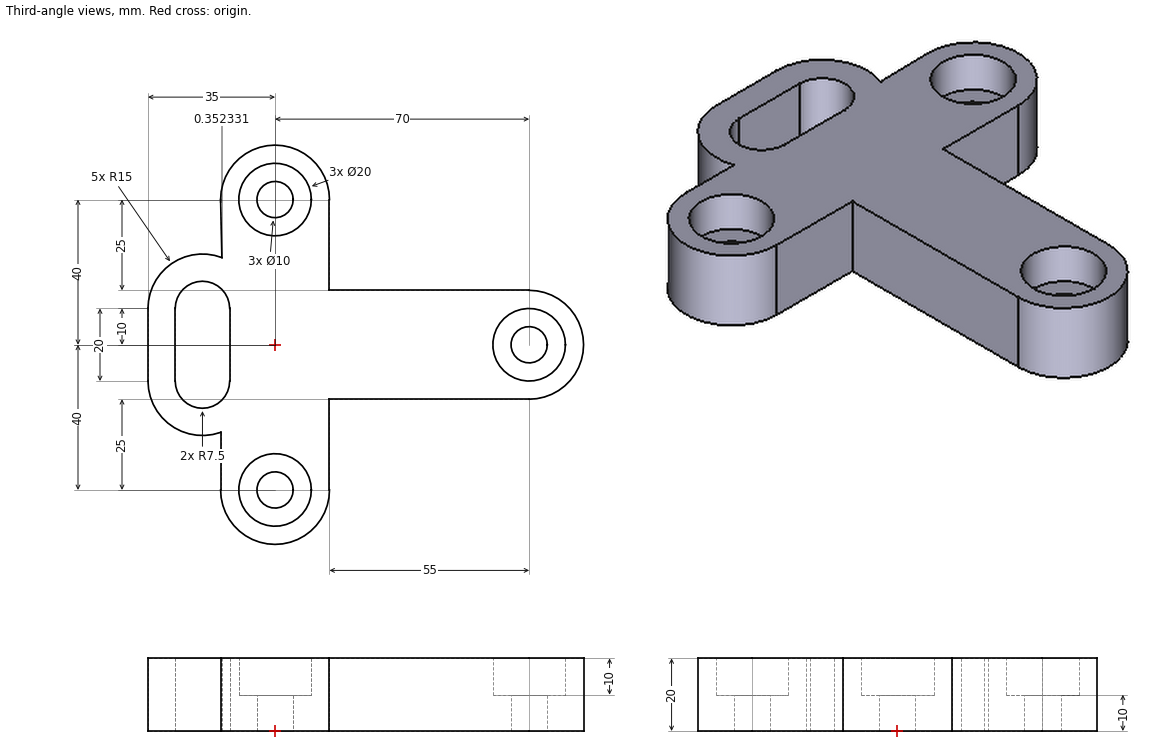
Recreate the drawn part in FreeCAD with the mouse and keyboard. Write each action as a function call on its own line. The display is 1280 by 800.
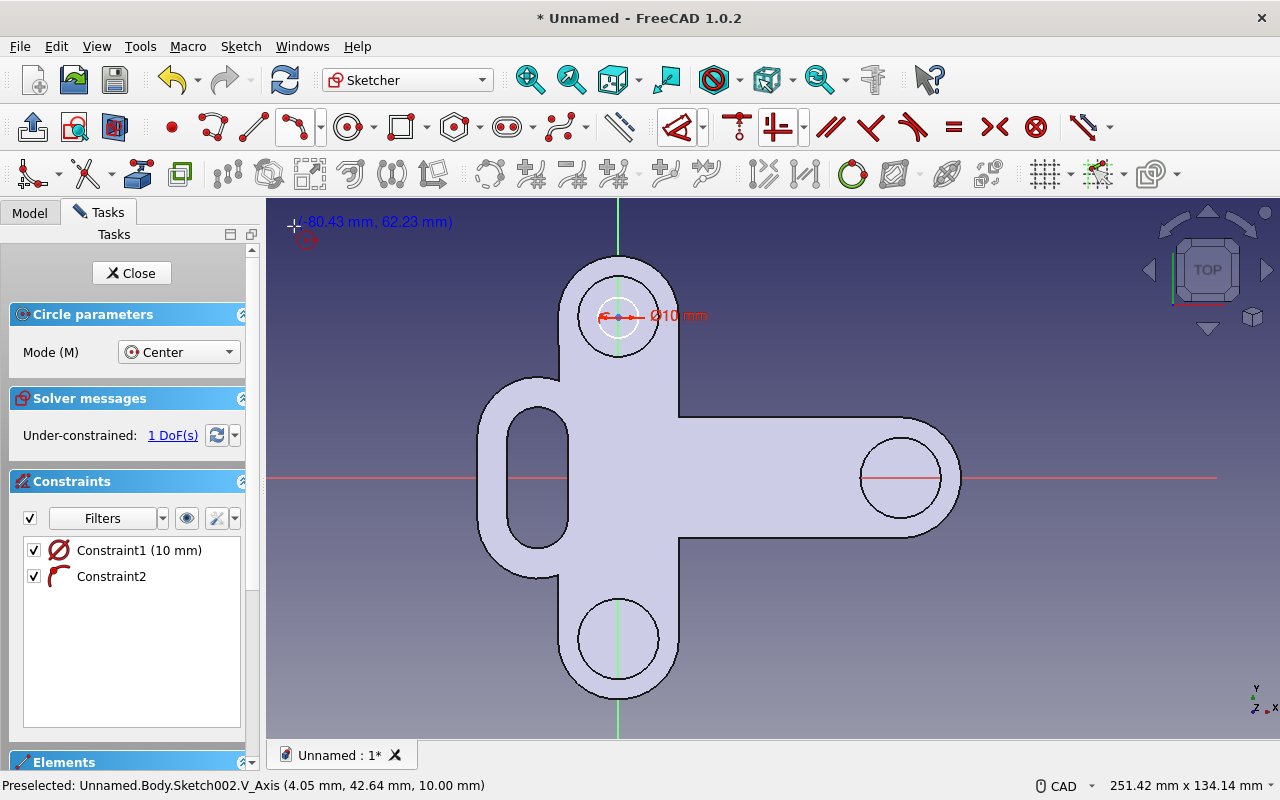
click(618, 639)
move(633, 625)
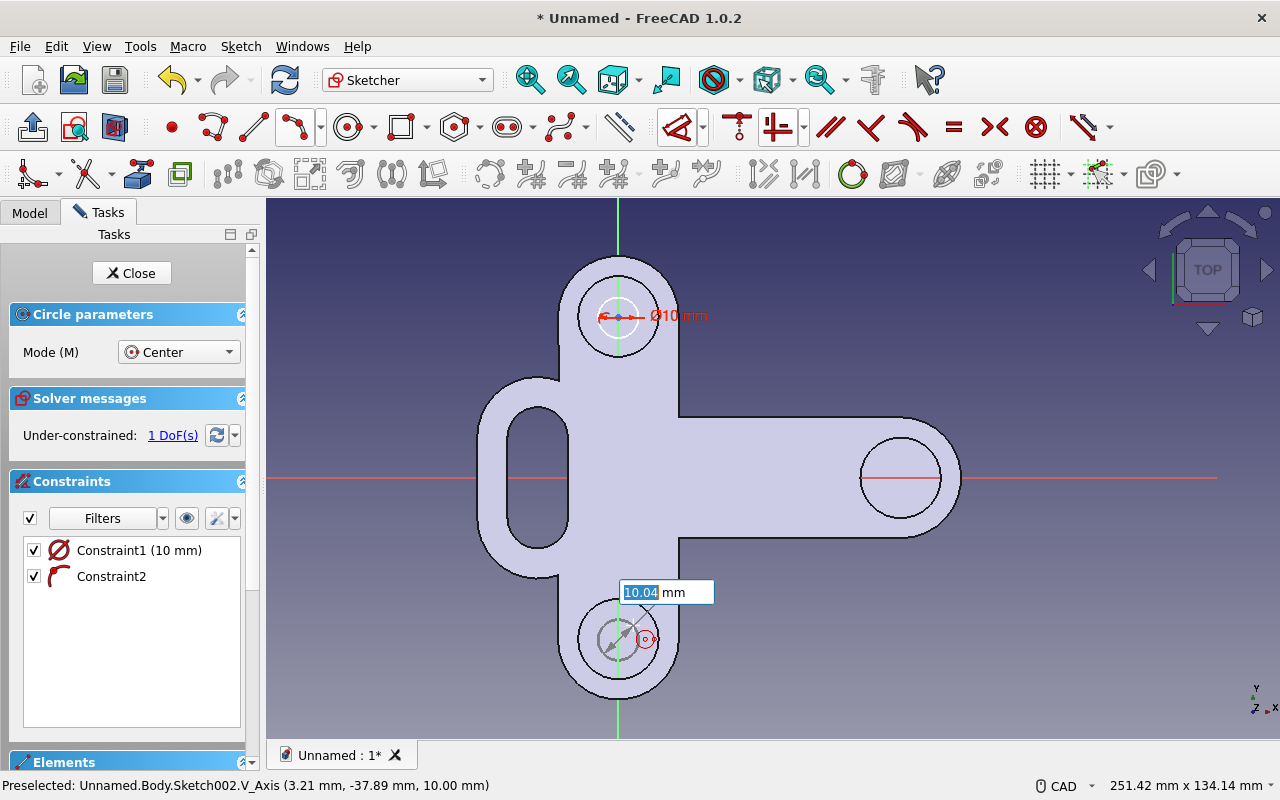
text(10)
key(Return)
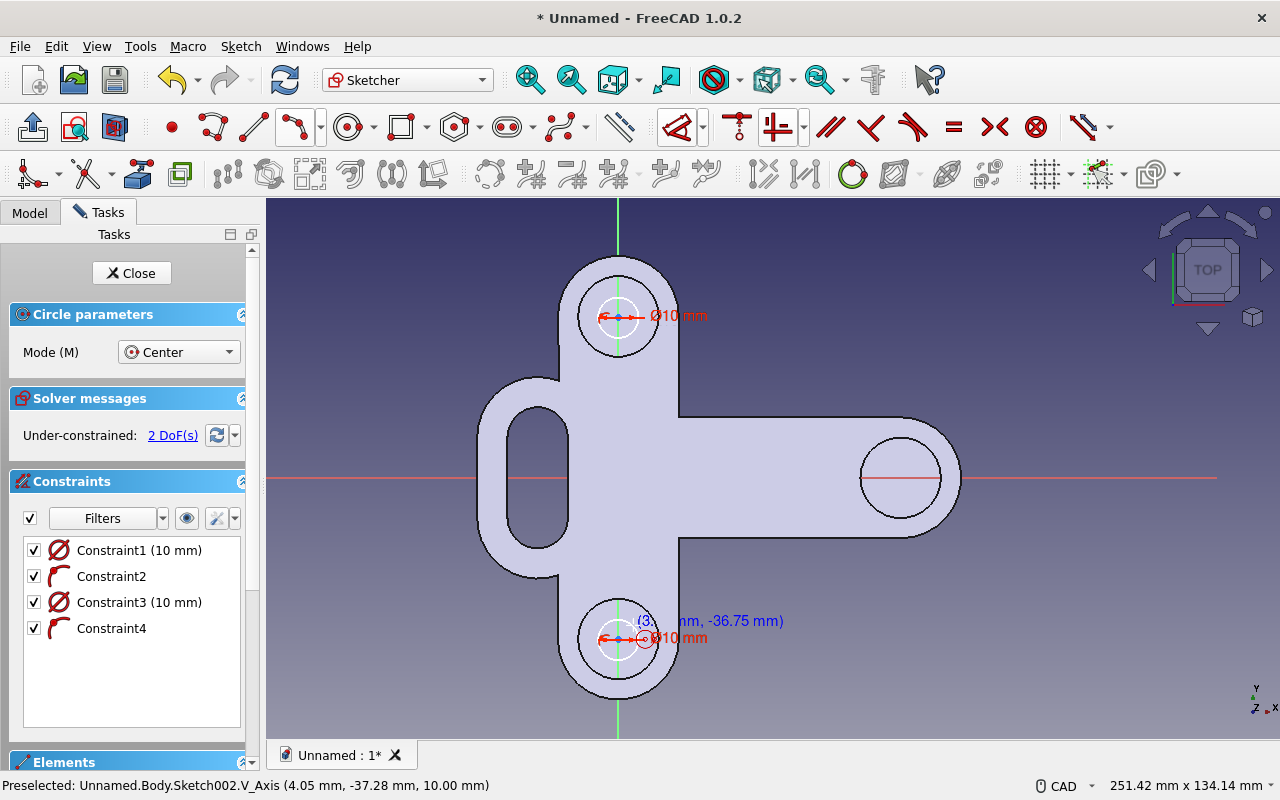
click(901, 478)
move(915, 464)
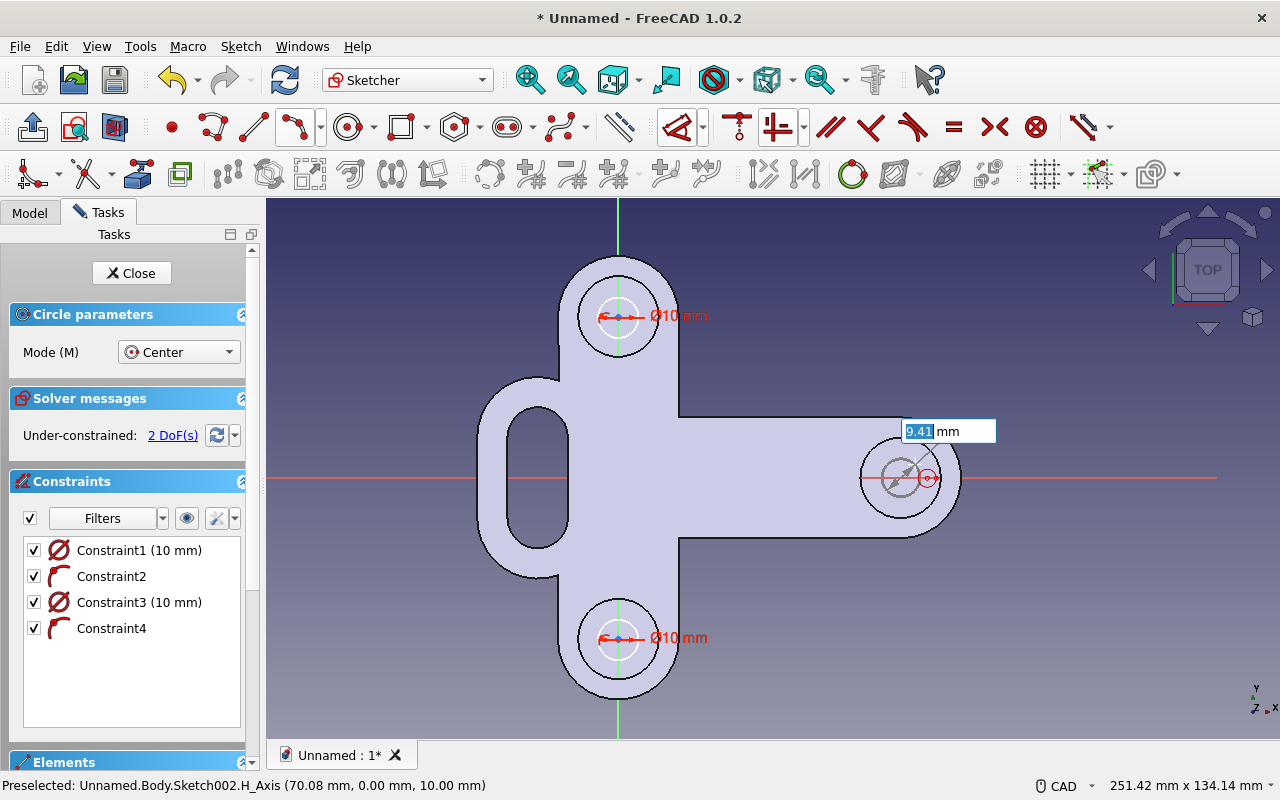
text(10)
key(Return)
key(Escape)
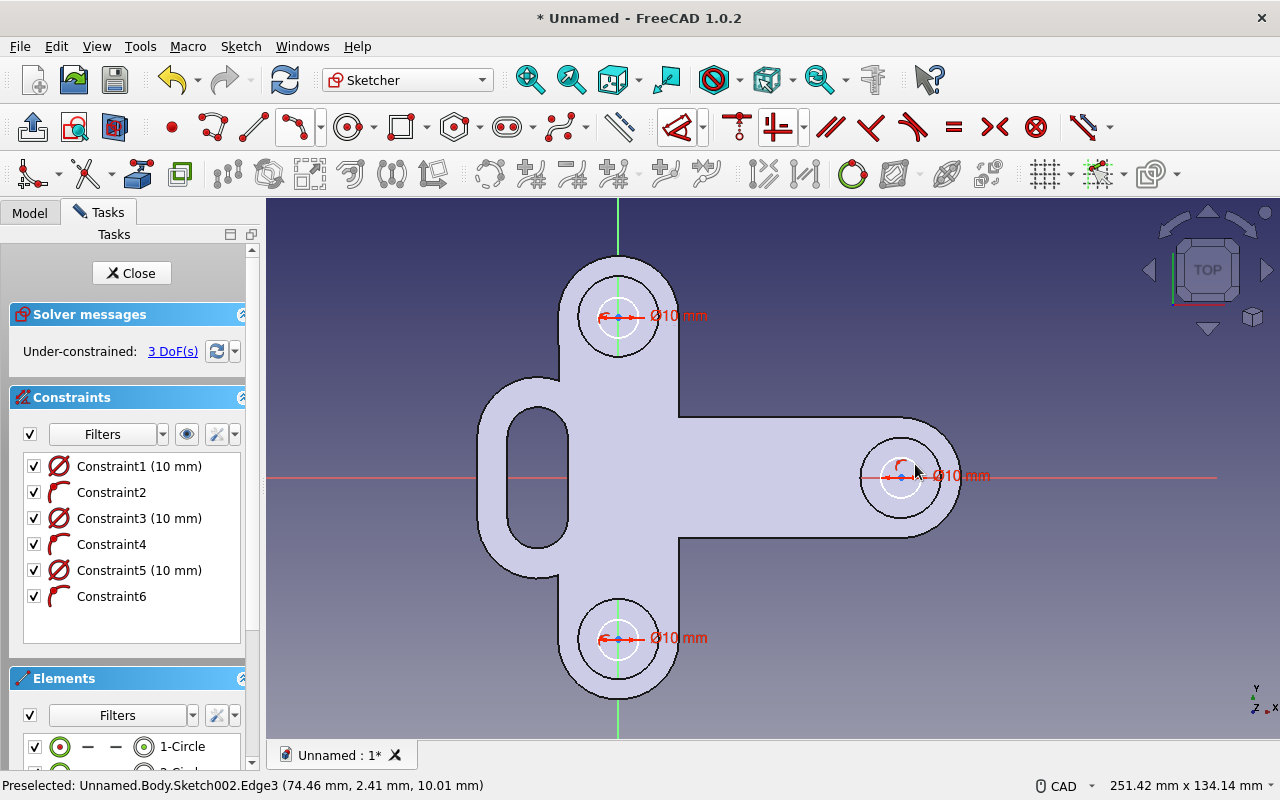
click(618, 318)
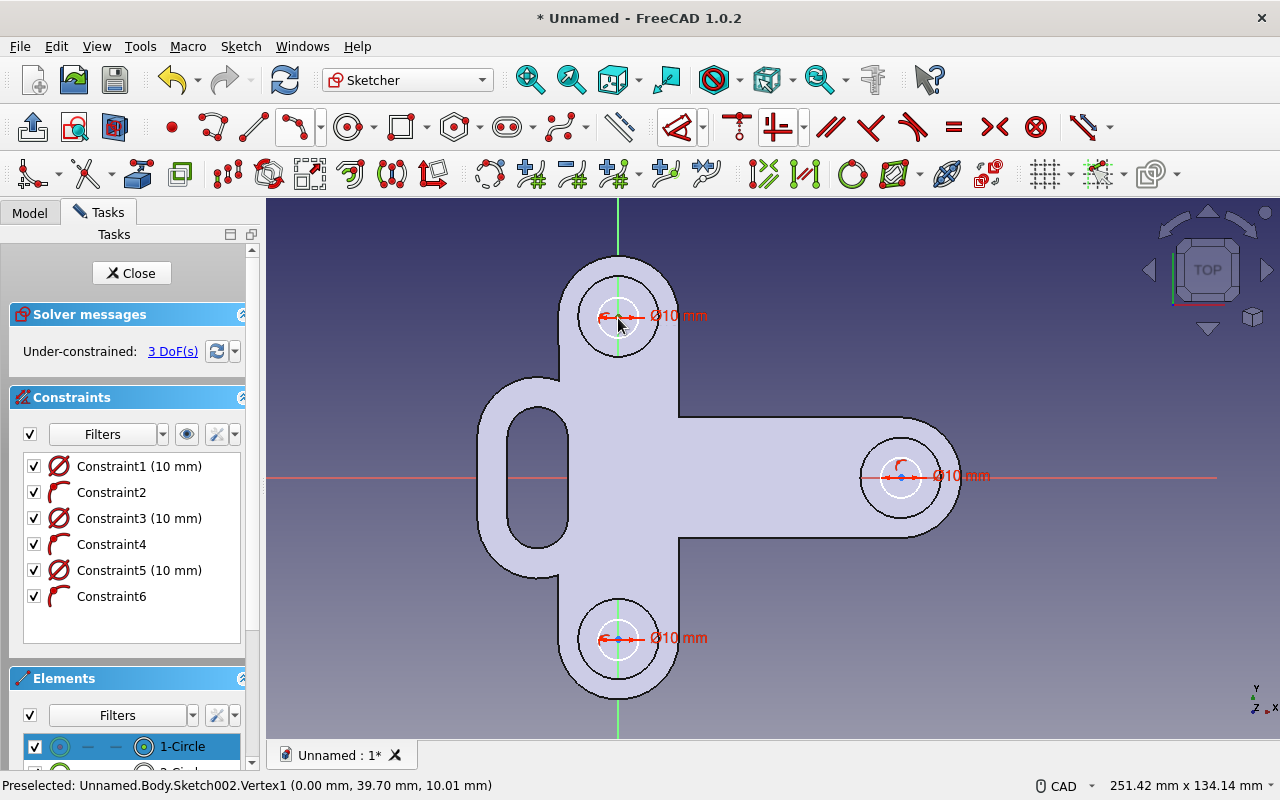
key(i)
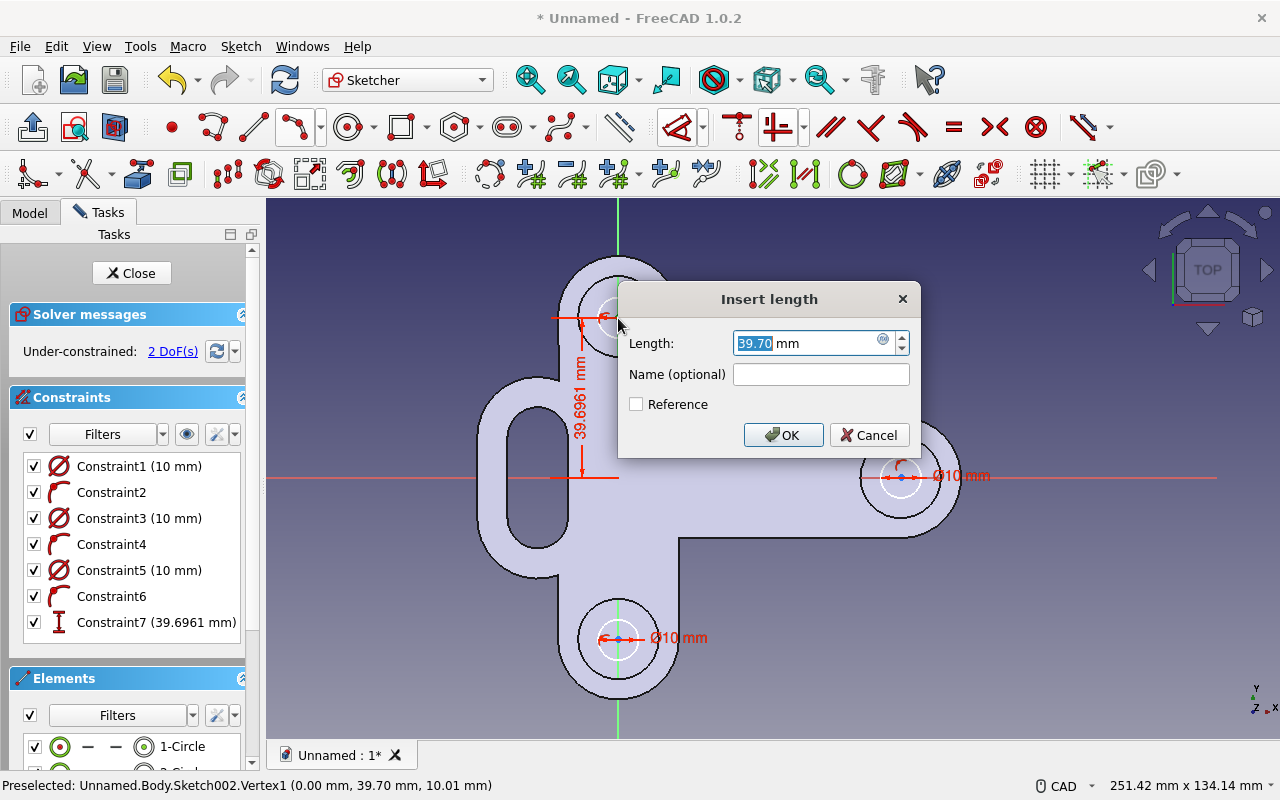
text(40)
key(Return)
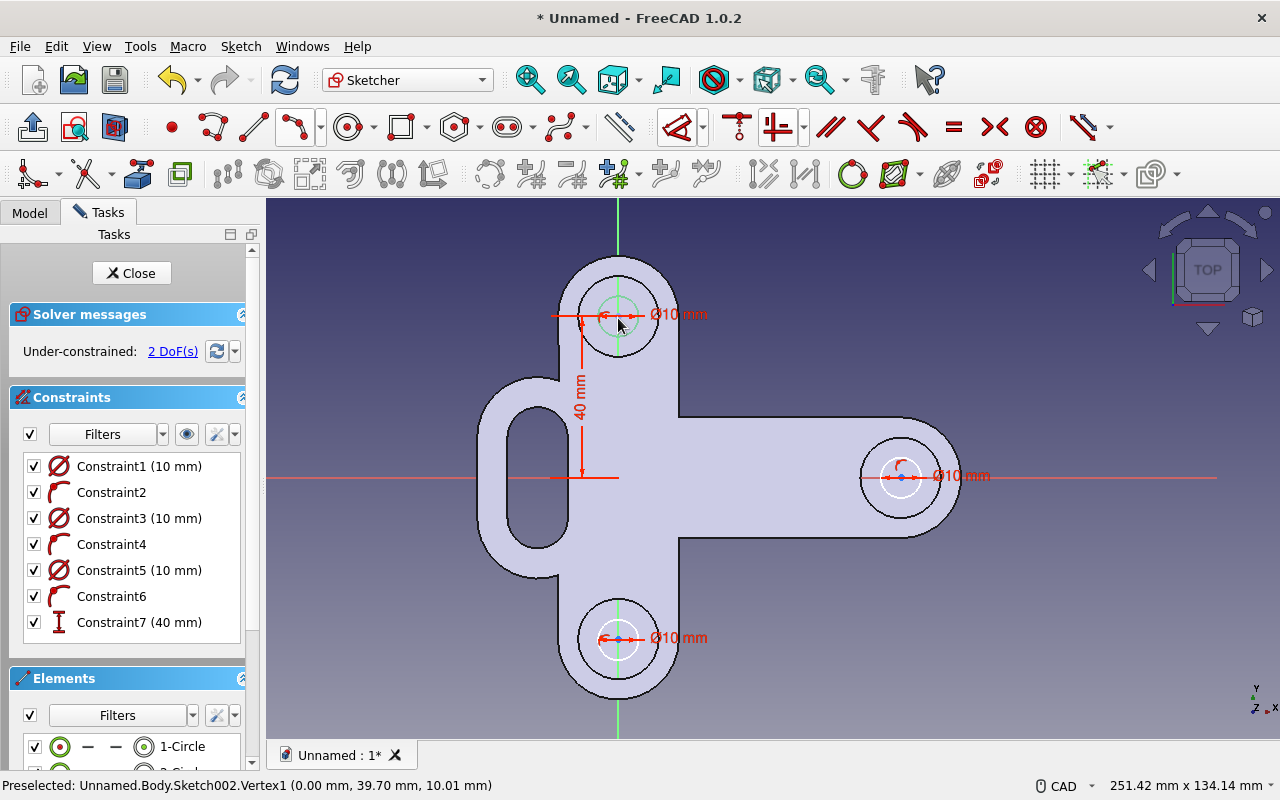
click(618, 640)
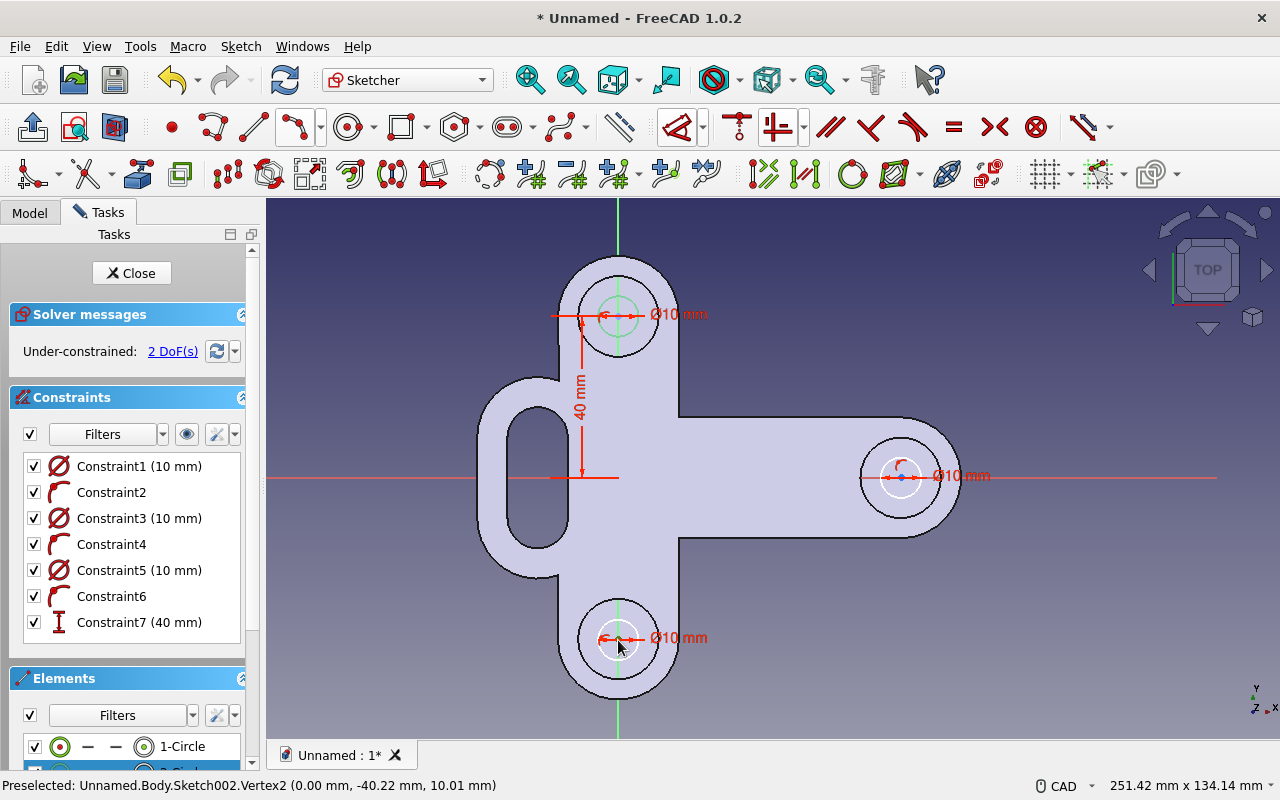
key(i)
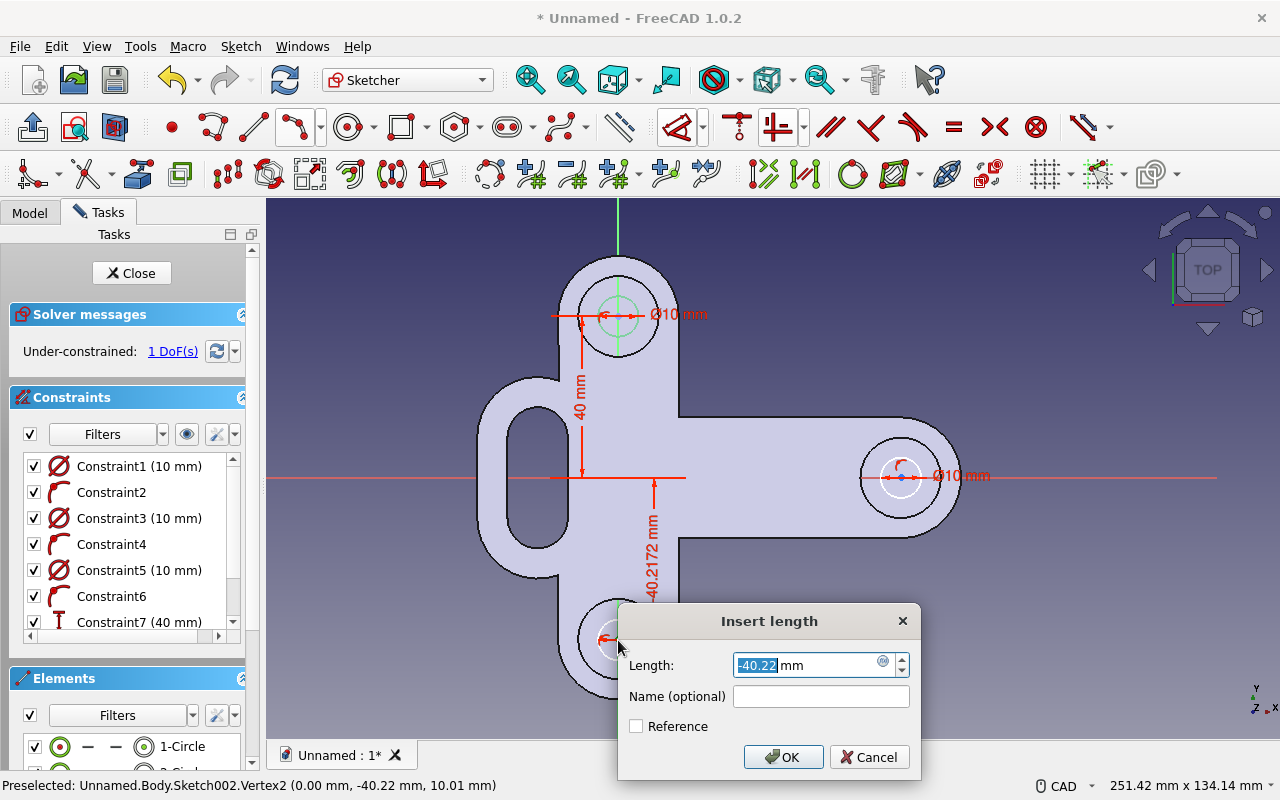
text(-40)
key(Return)